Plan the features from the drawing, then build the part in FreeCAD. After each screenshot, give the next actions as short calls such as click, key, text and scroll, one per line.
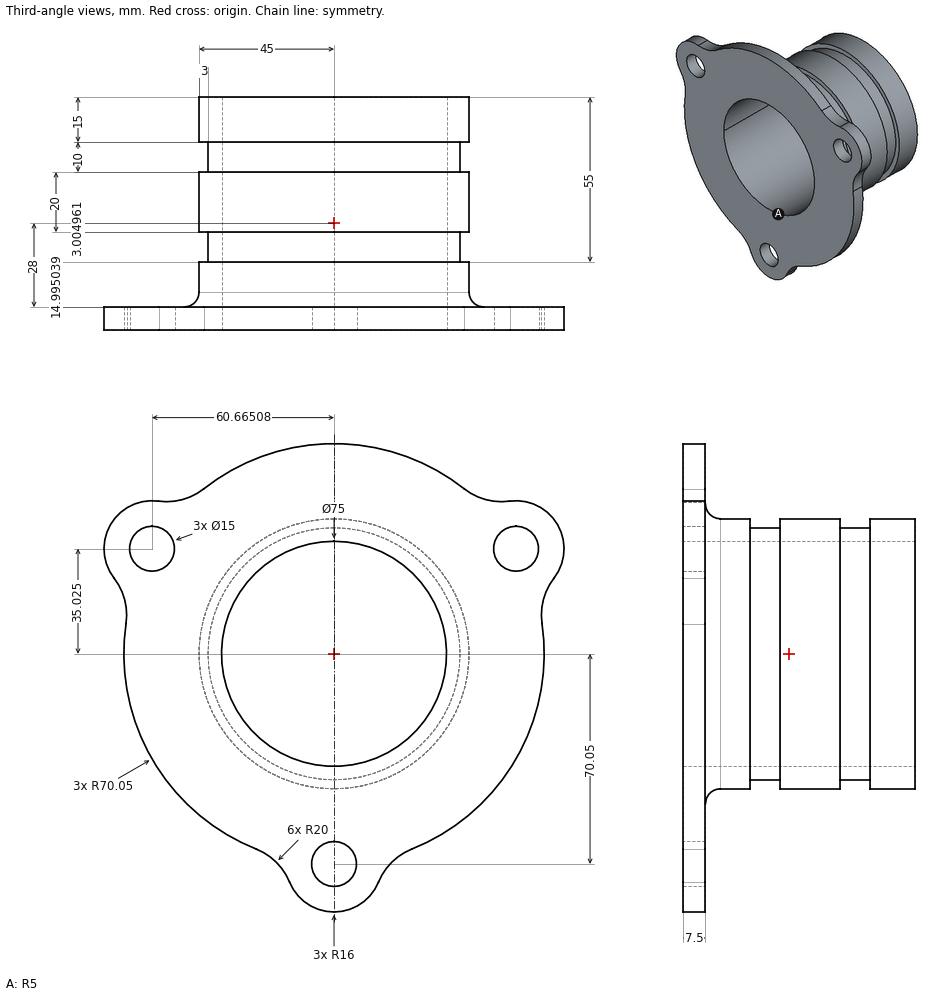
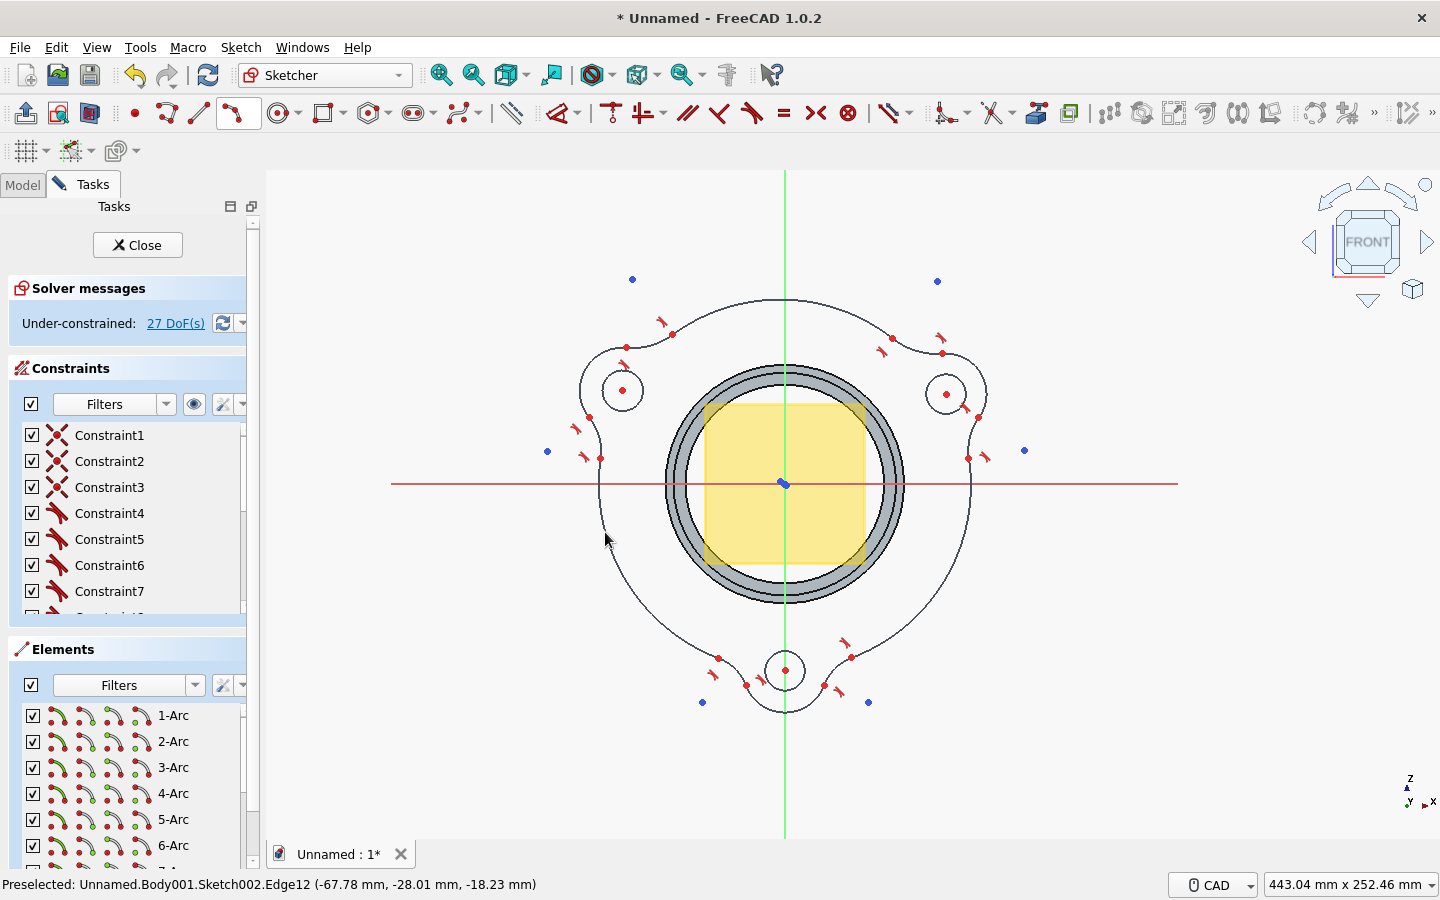
click(830, 307)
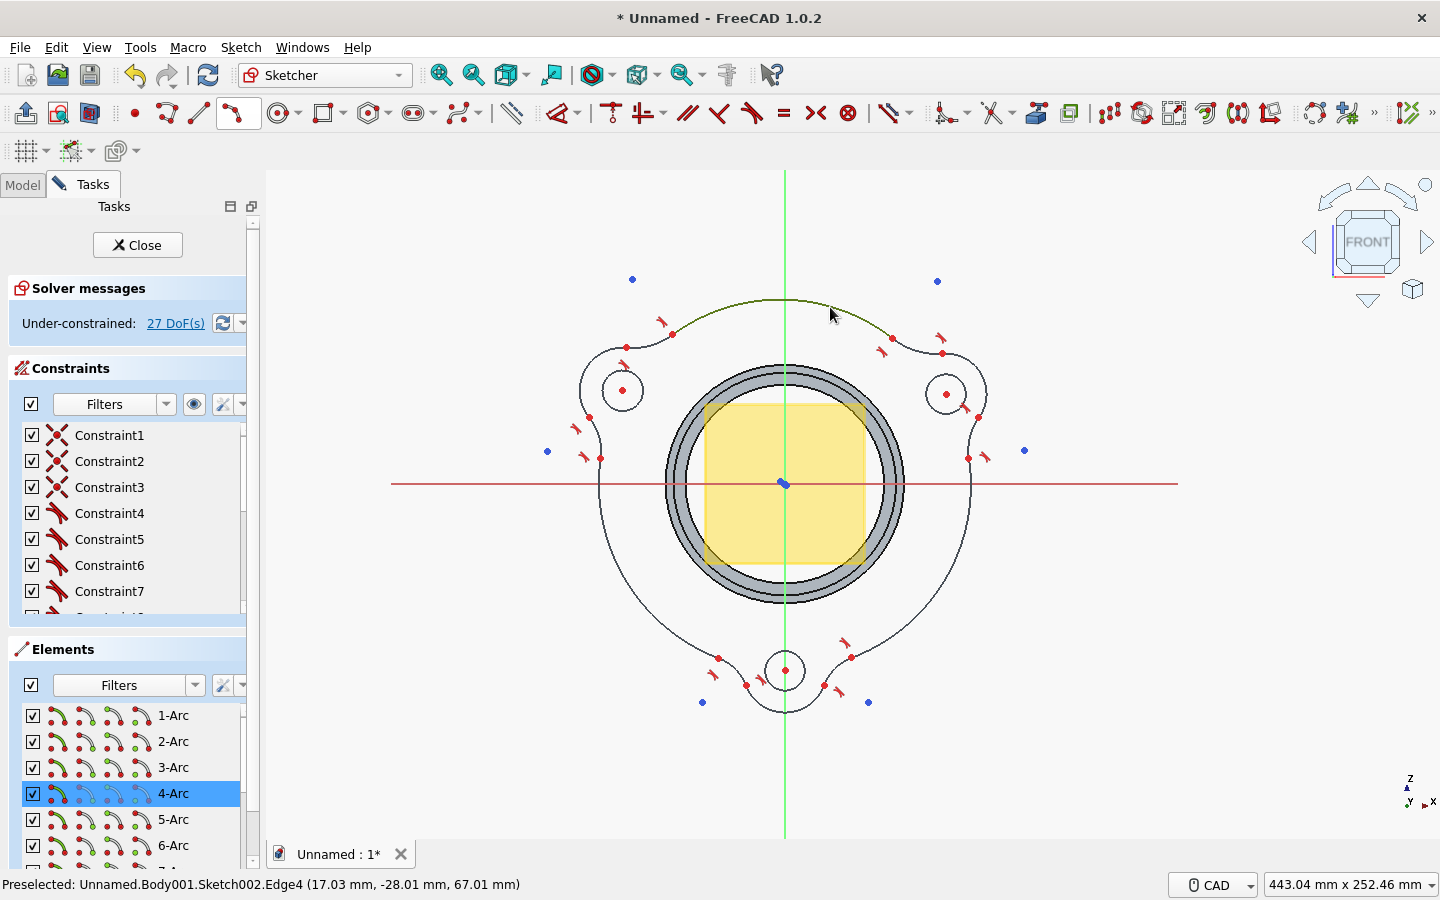
click(915, 618)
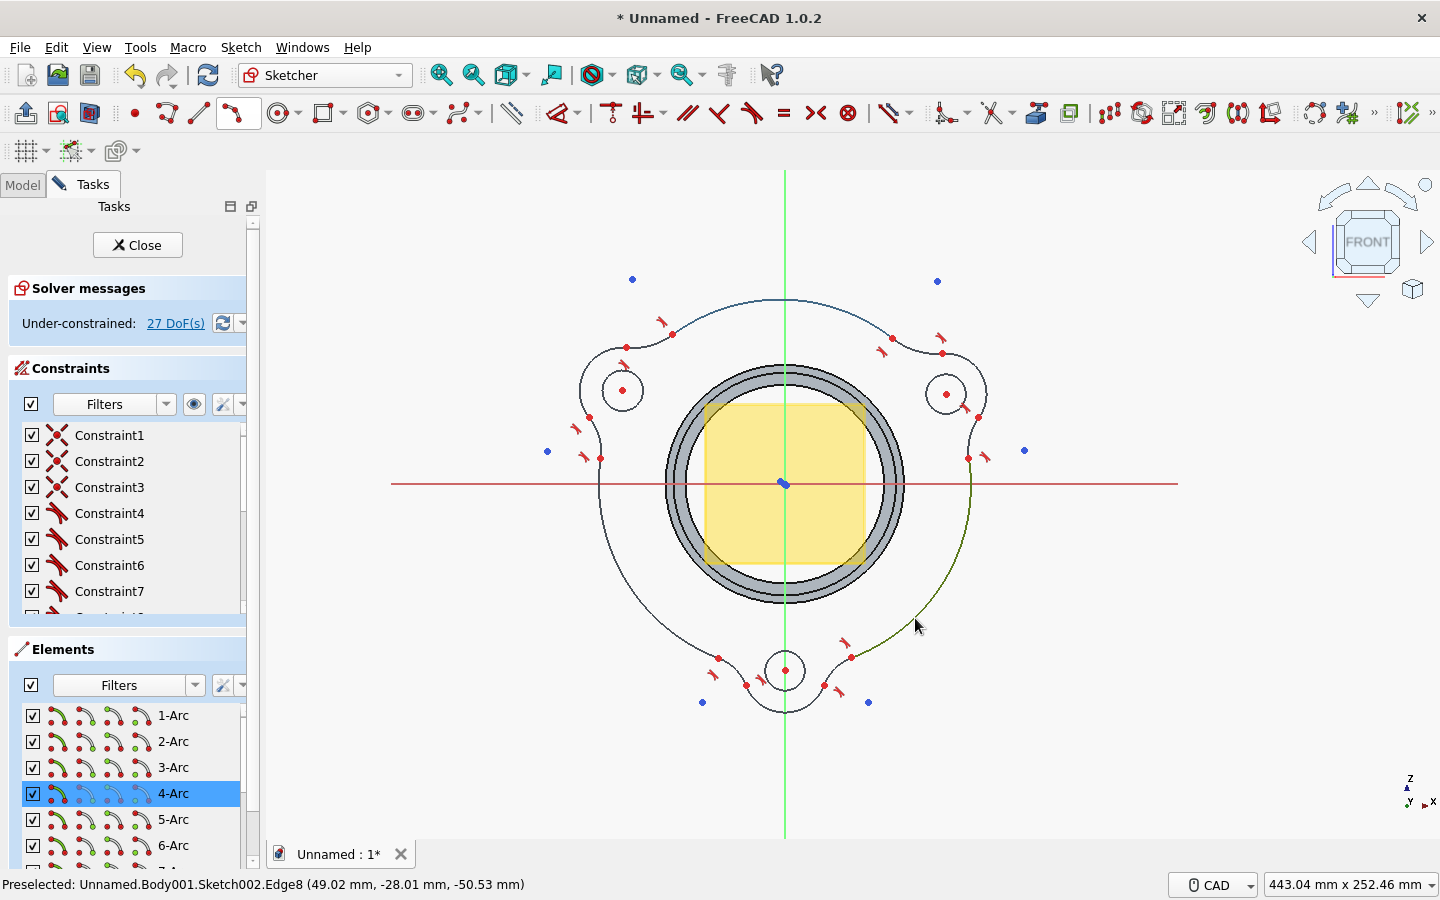
key(c)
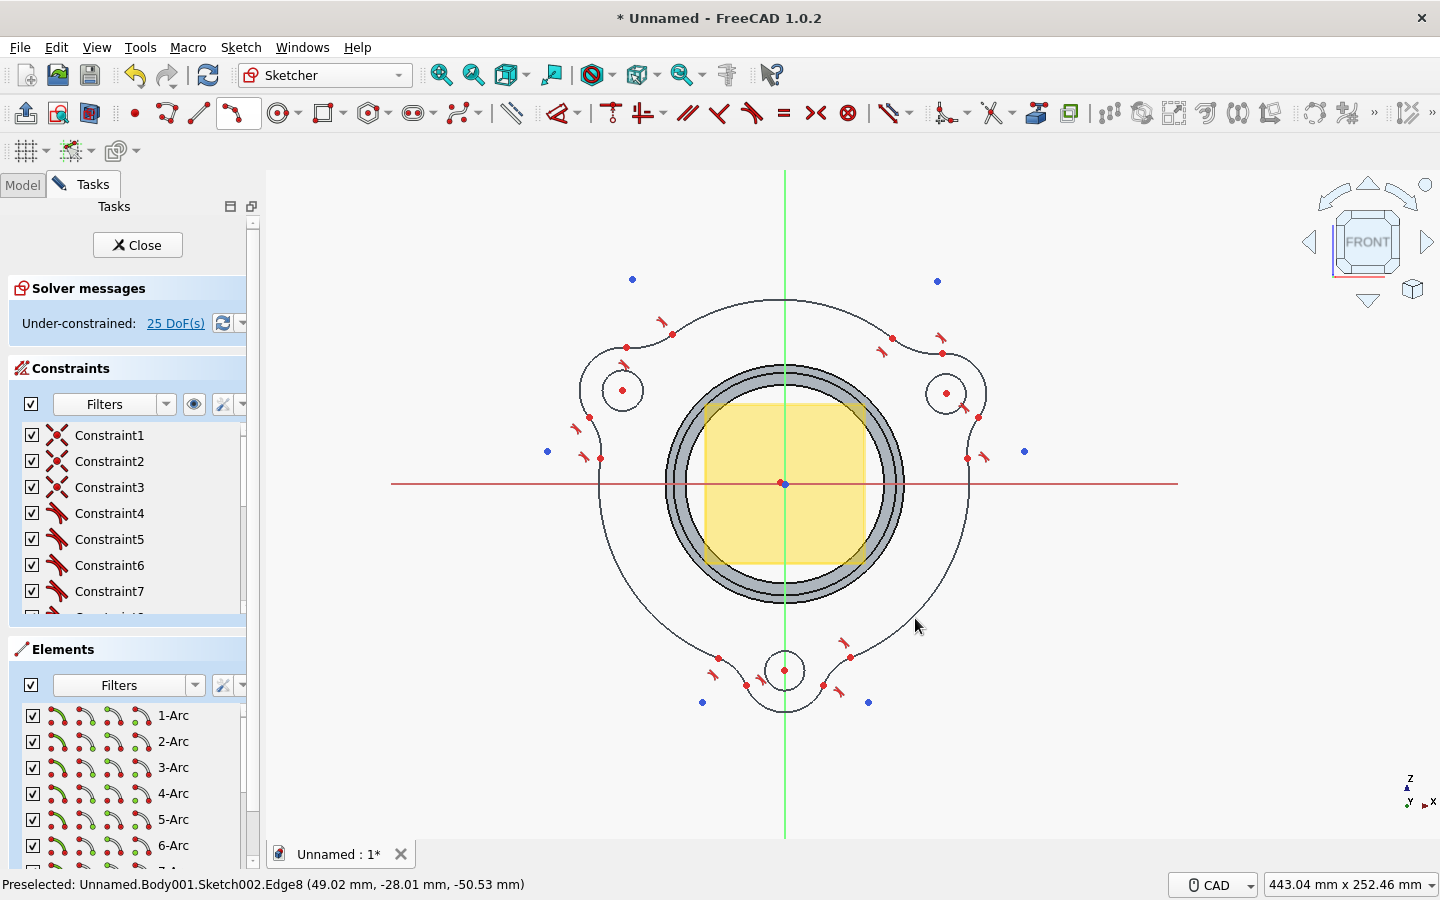
click(830, 307)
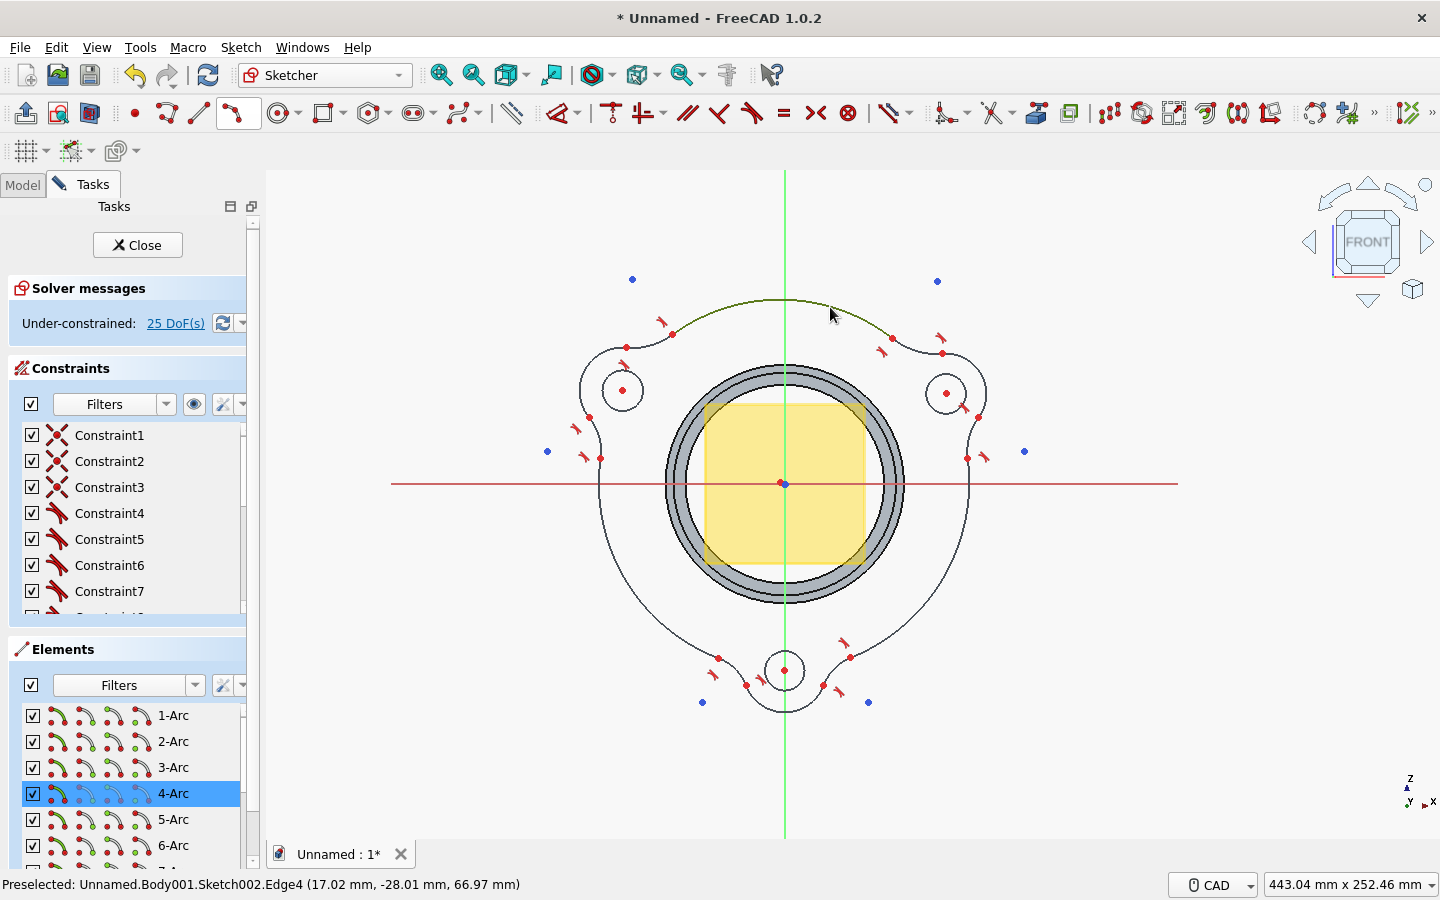
click(605, 533)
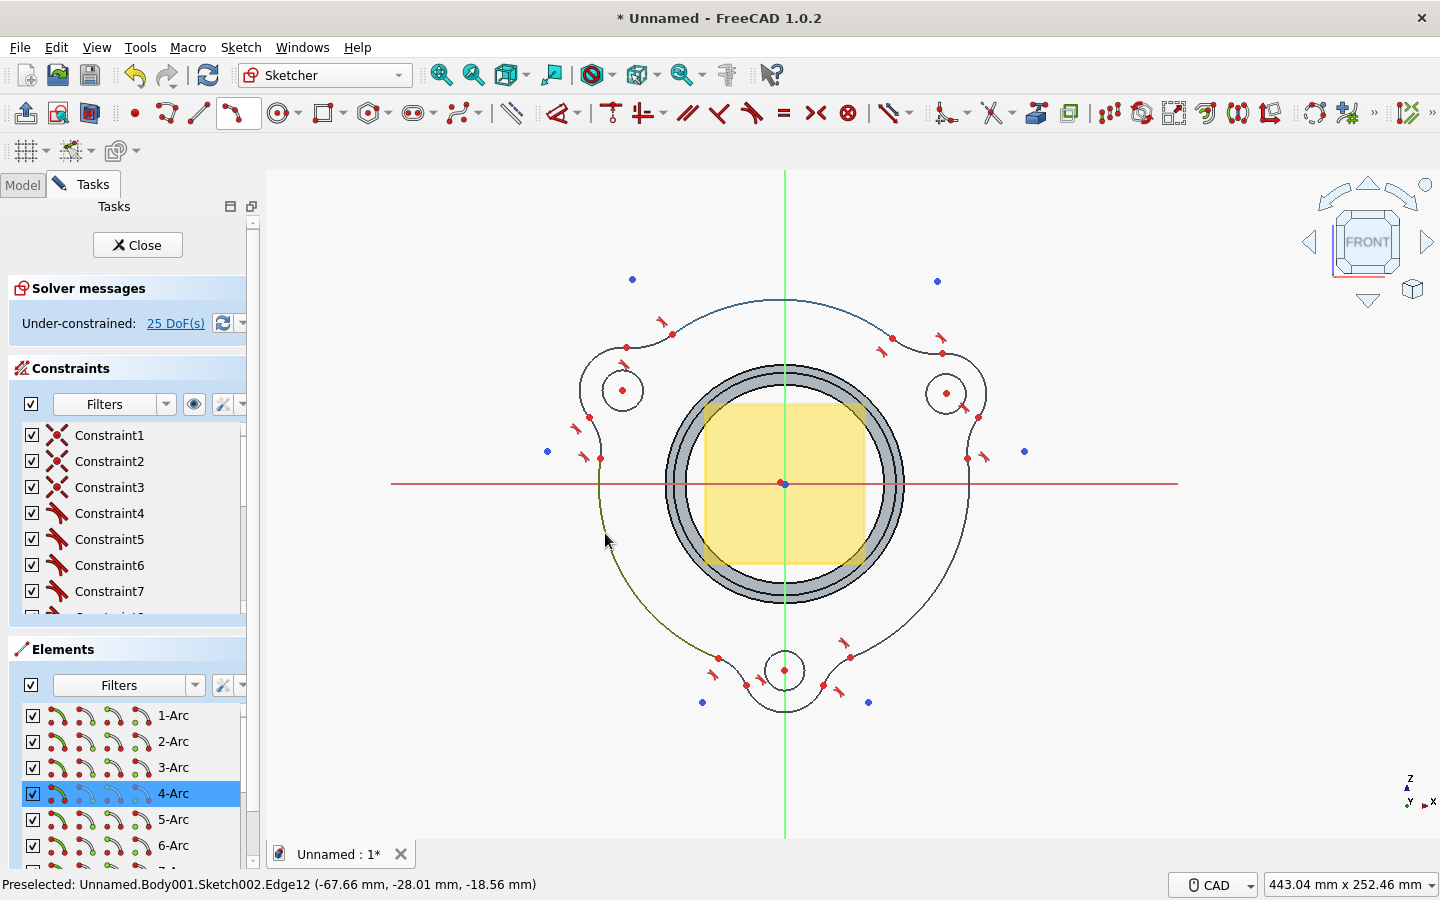
click(612, 114)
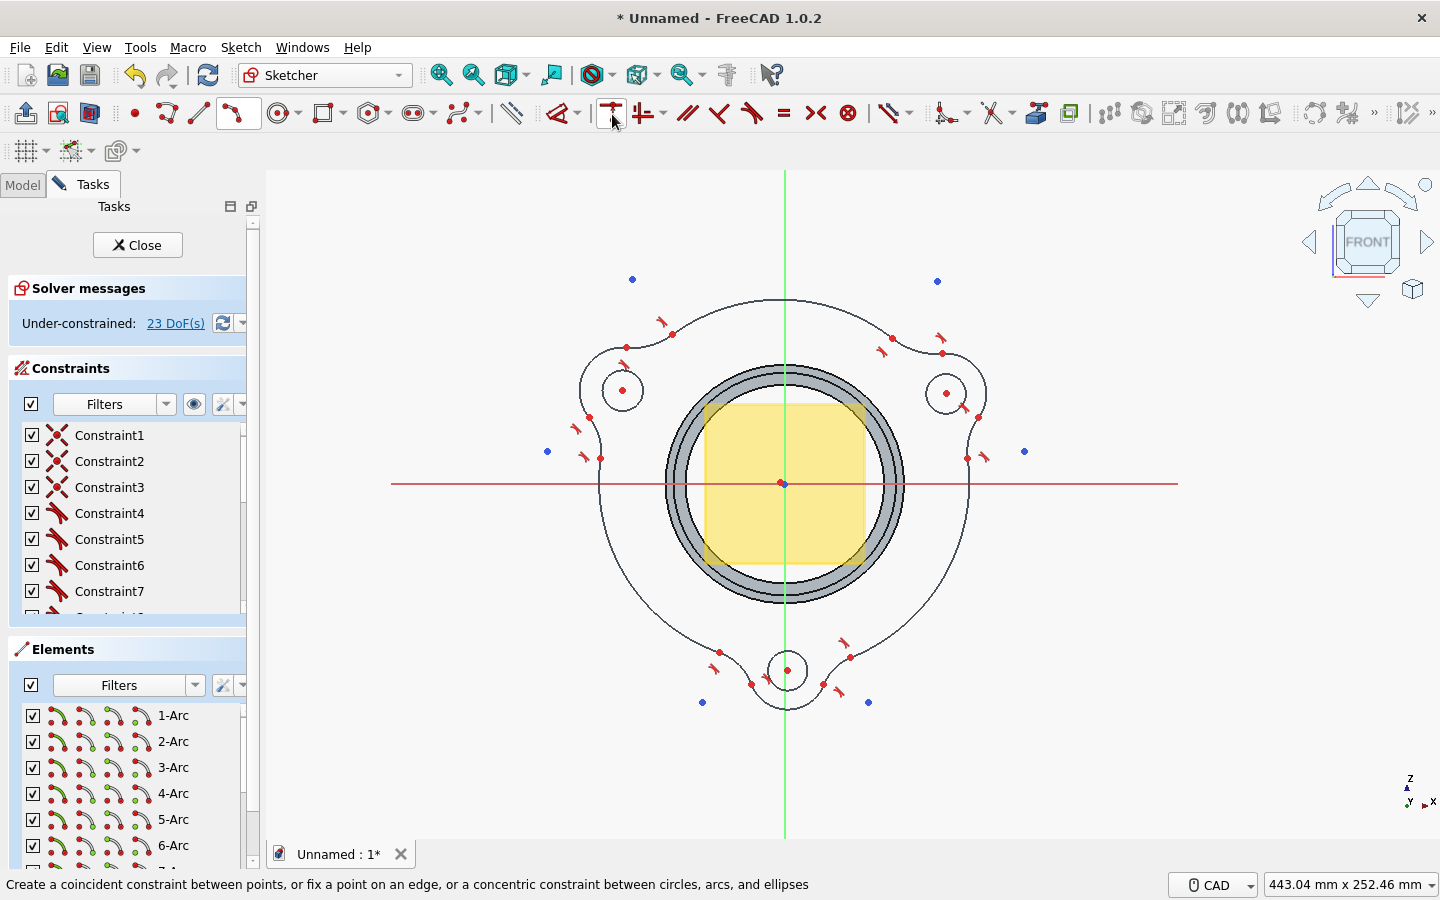
scroll(782, 483, up, 4)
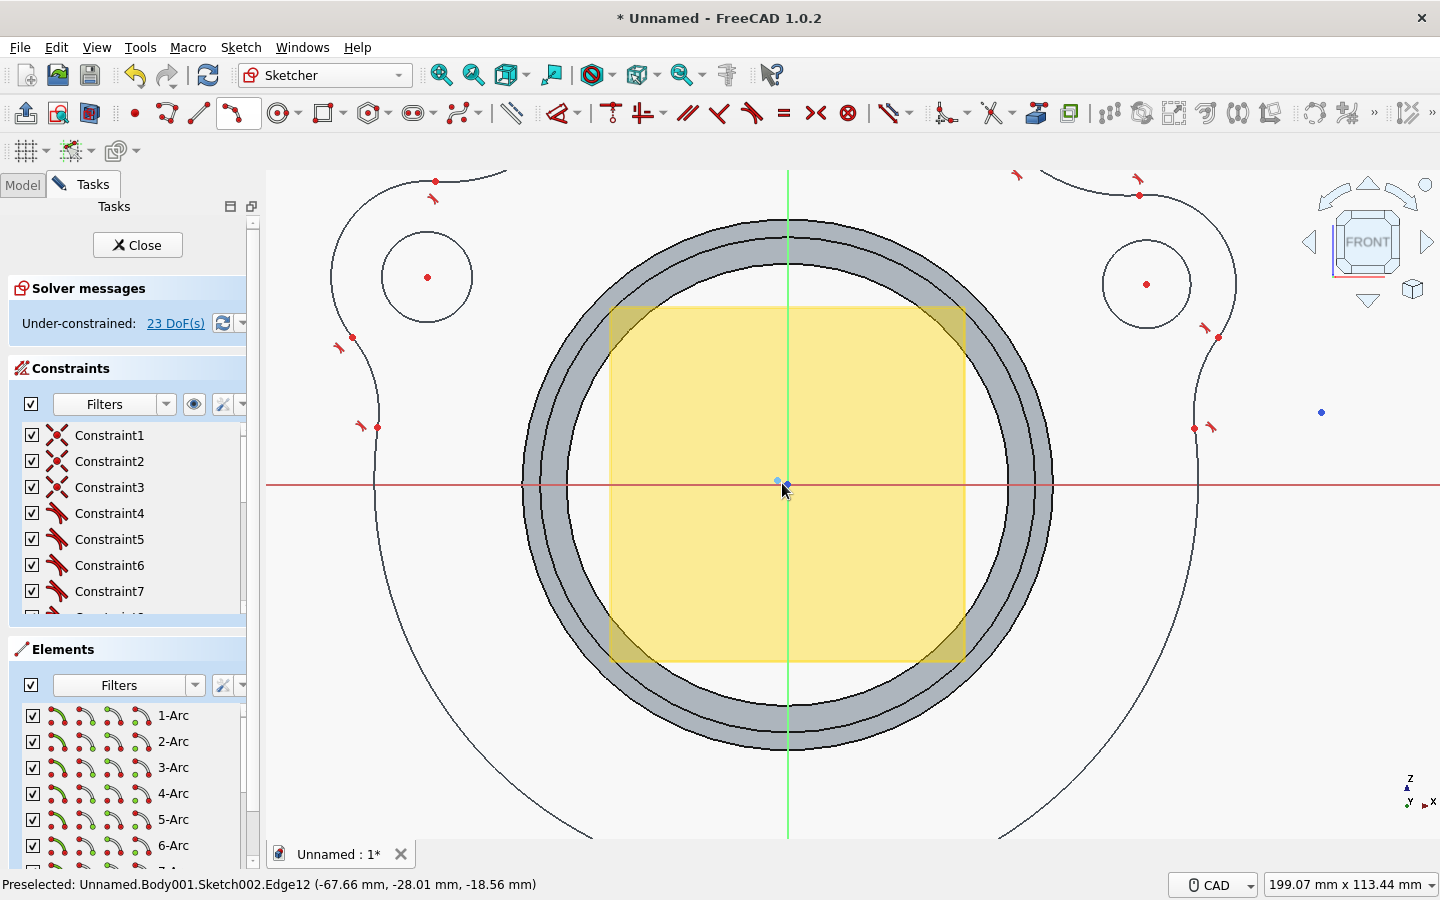
drag(767, 471, 798, 495)